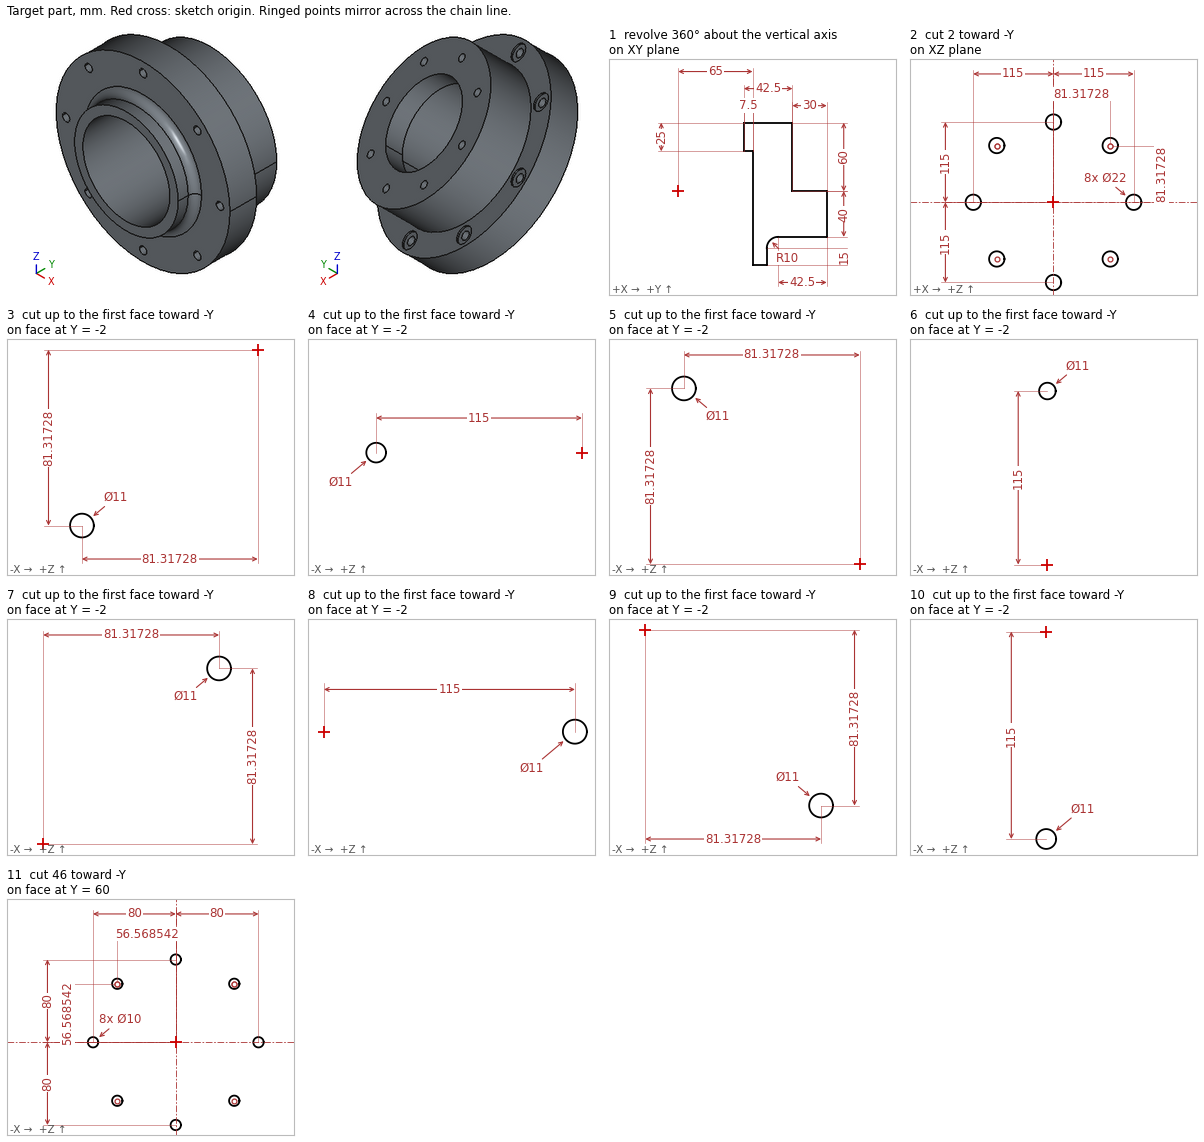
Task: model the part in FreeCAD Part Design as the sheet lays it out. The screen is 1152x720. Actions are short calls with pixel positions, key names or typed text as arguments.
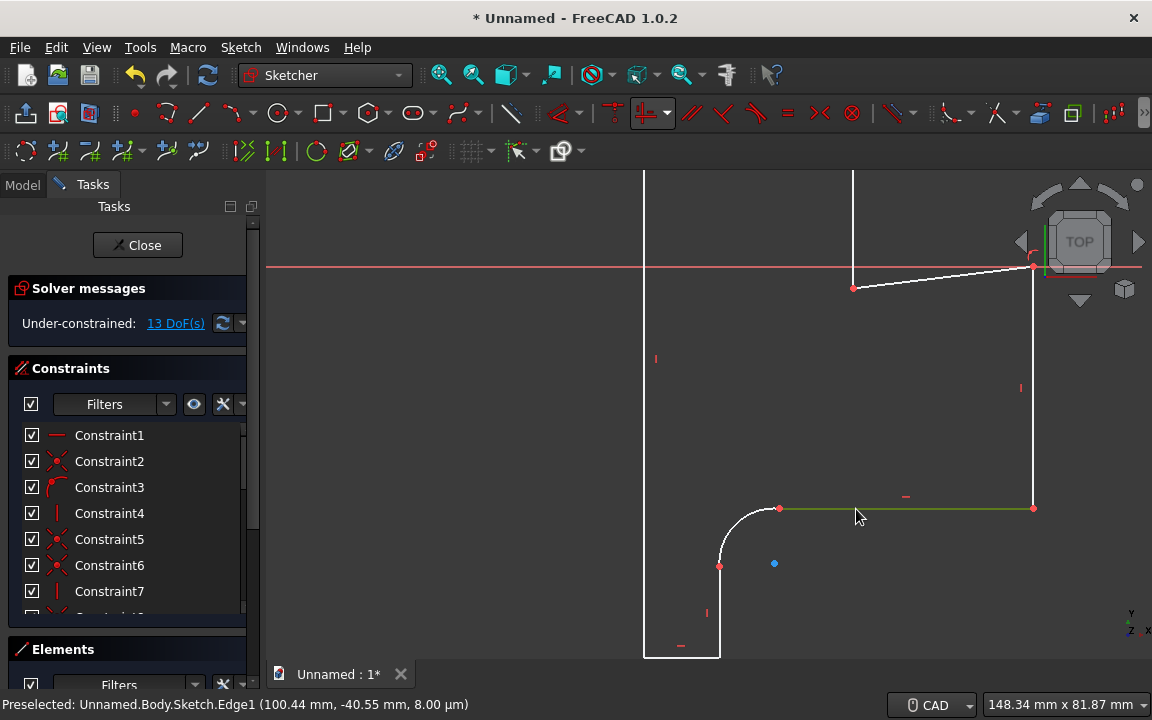
click(752, 513)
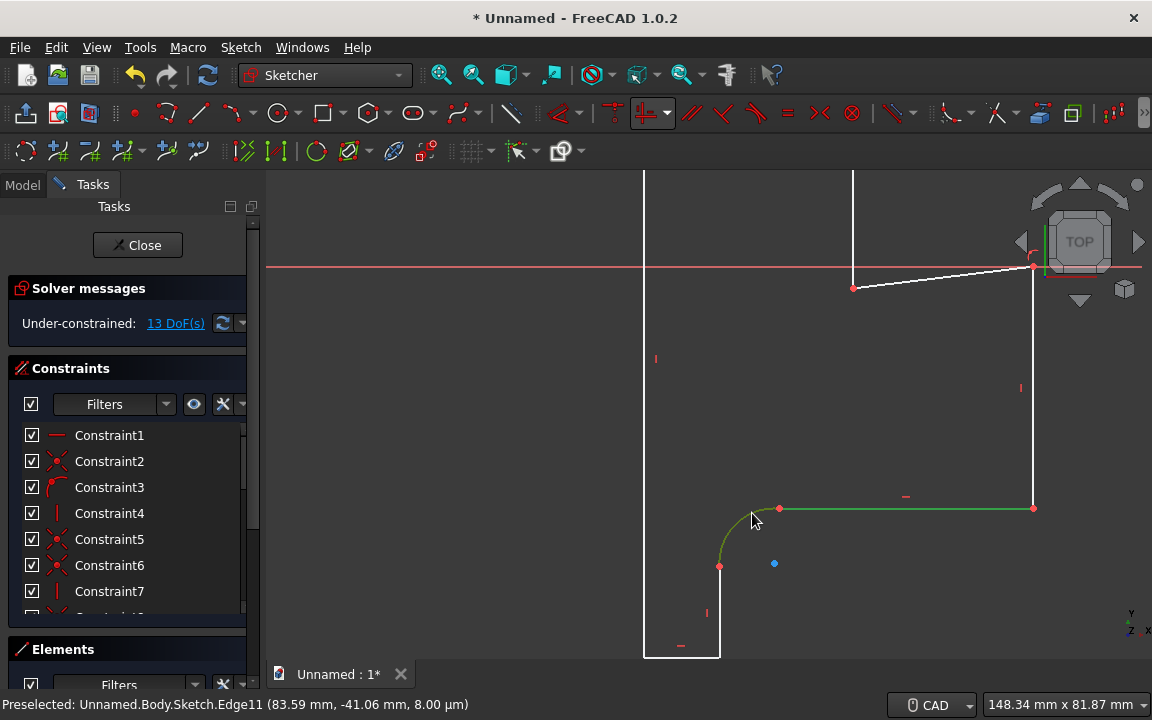
key(t)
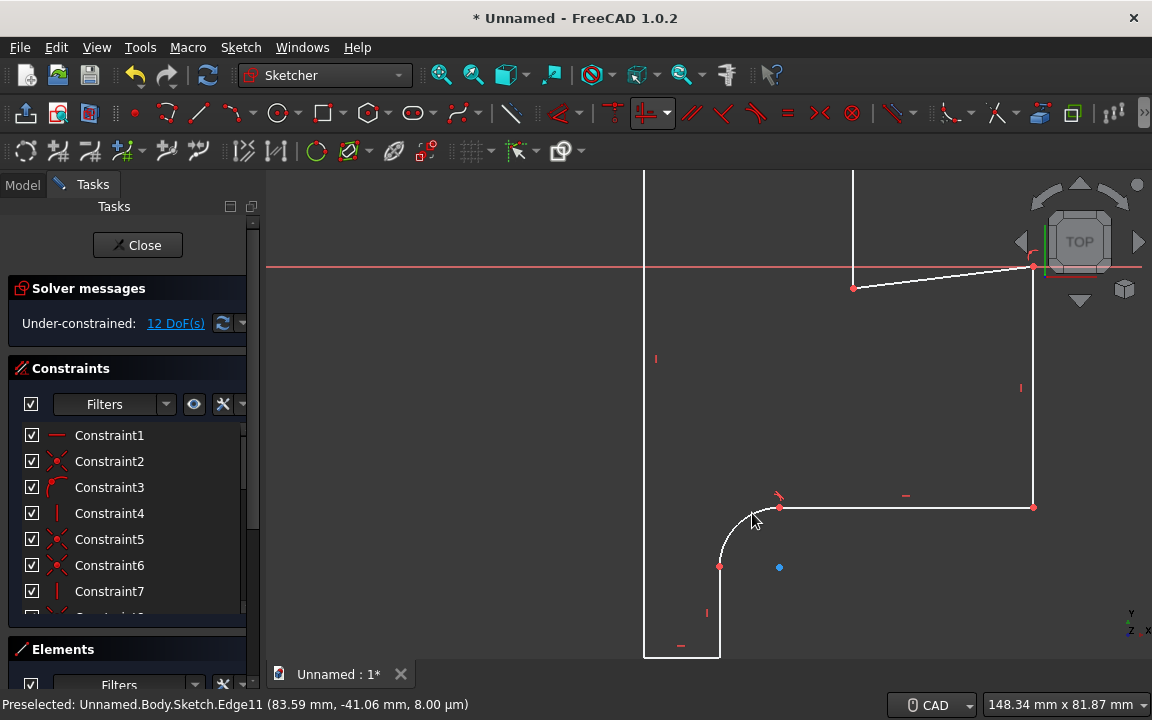
click(720, 630)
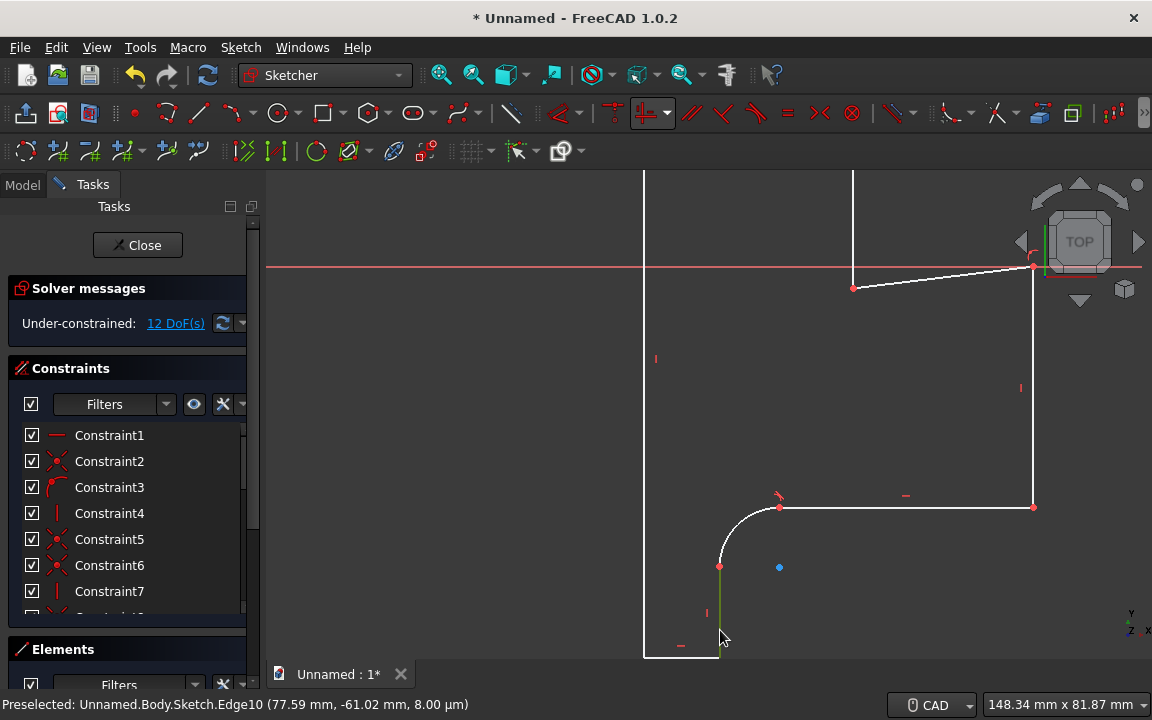
click(753, 514)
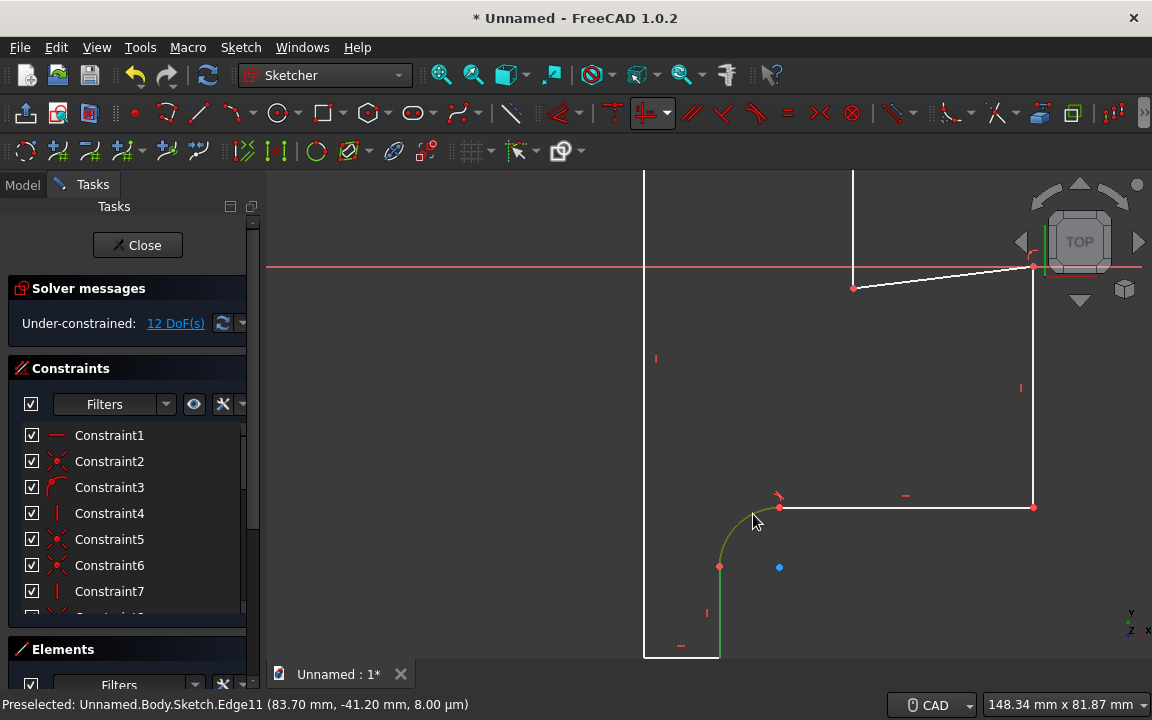
click(756, 114)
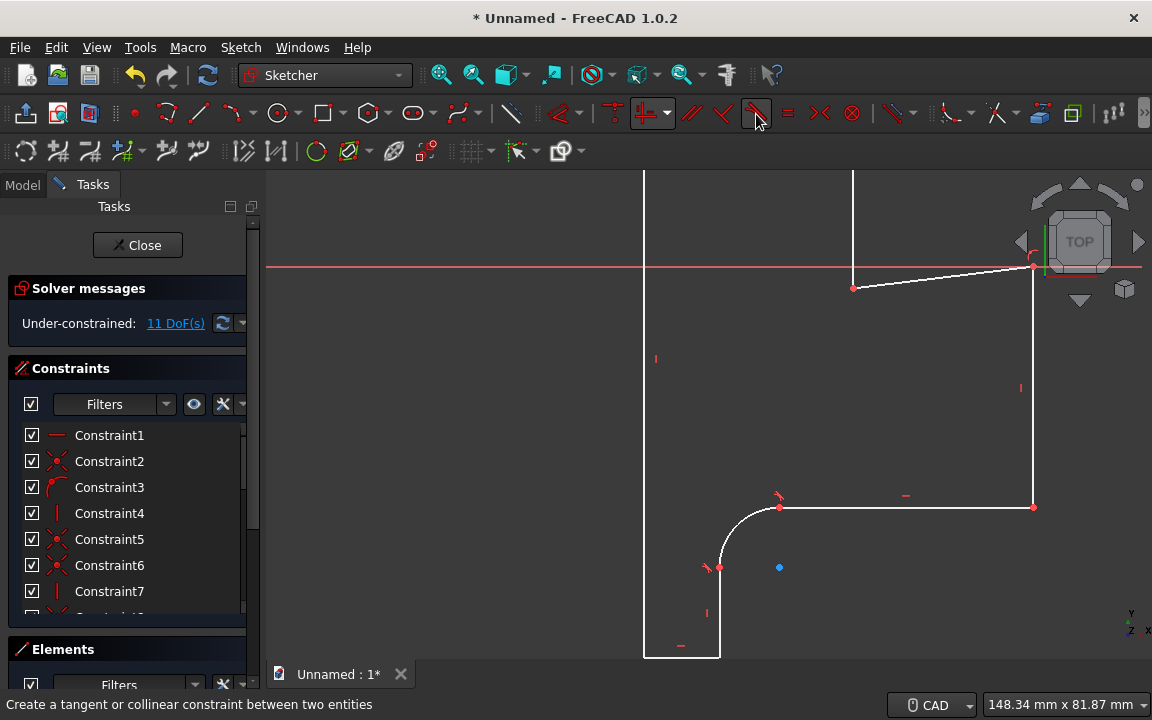
click(907, 282)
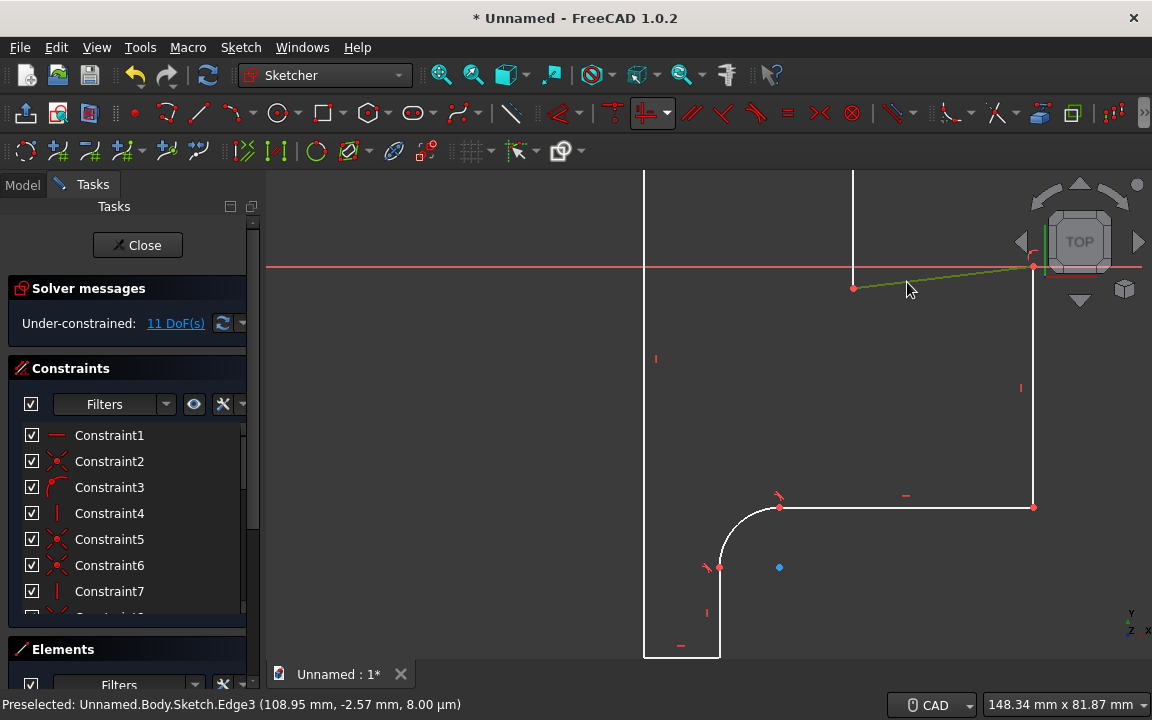
key(h)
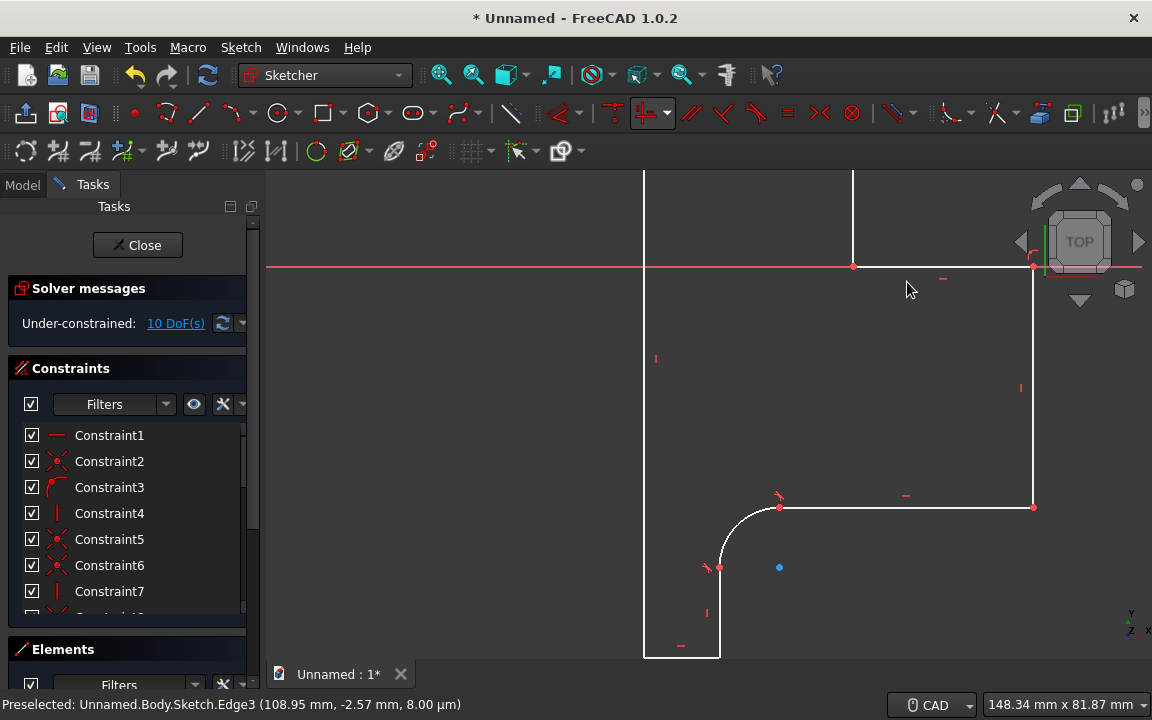
click(558, 114)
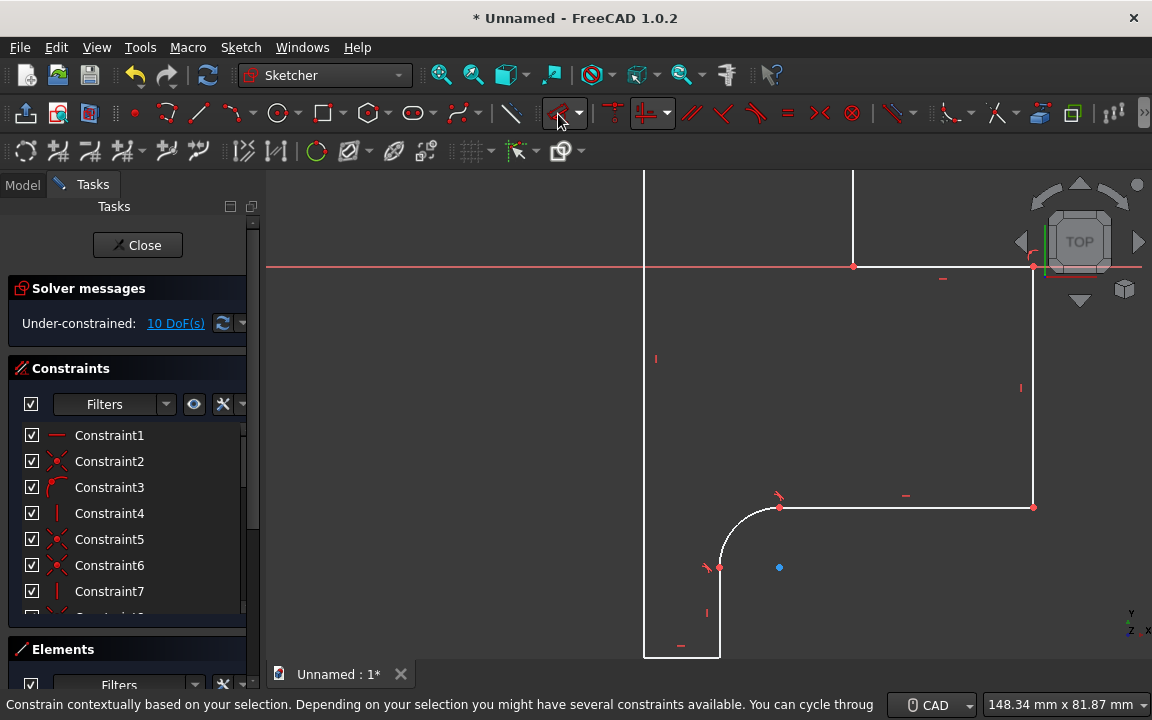
click(752, 514)
click(737, 486)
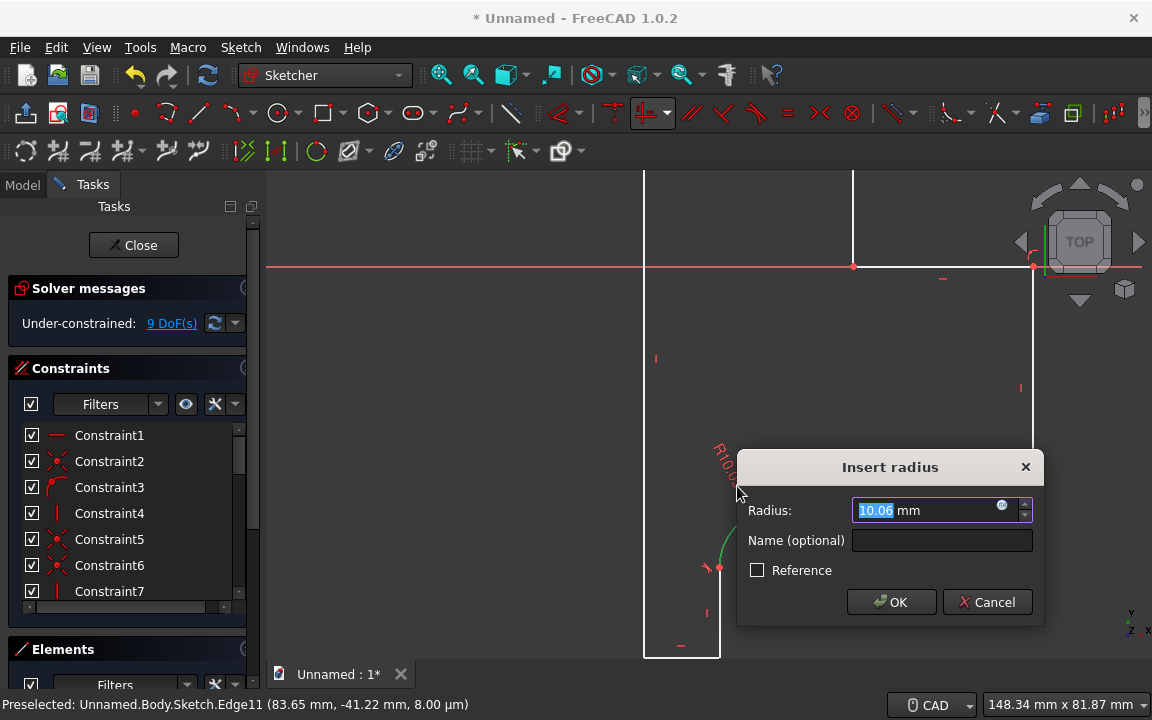
text(10)
key(Return)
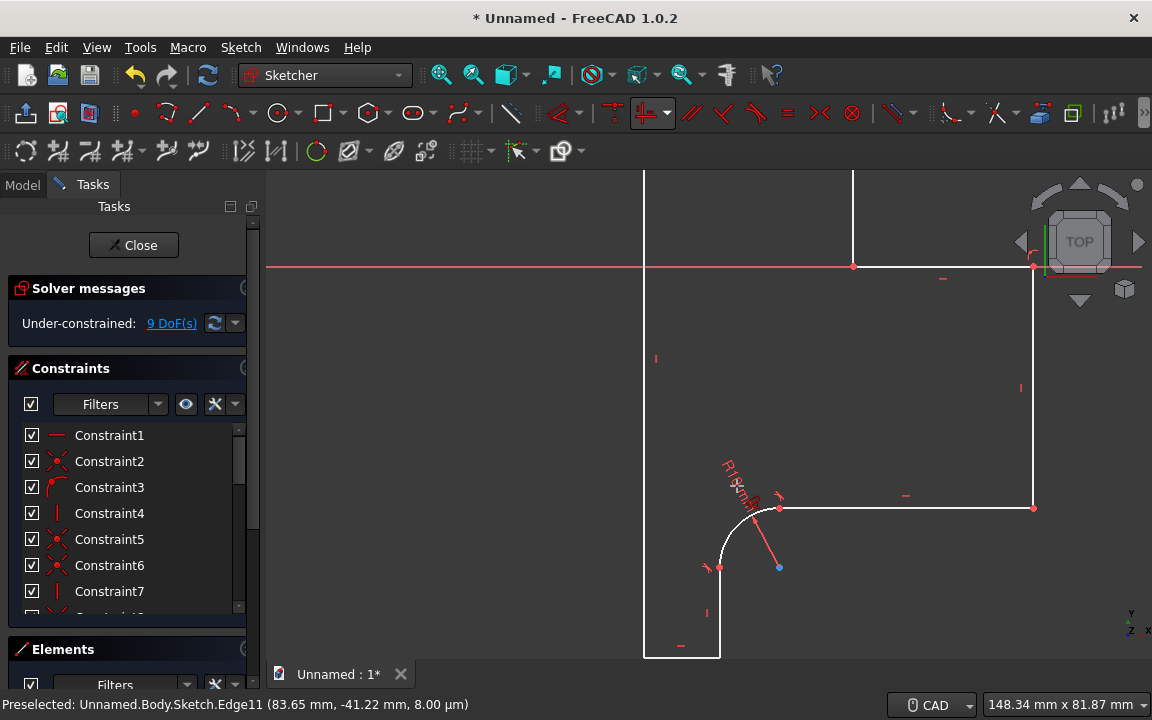
scroll(637, 523, down, 4)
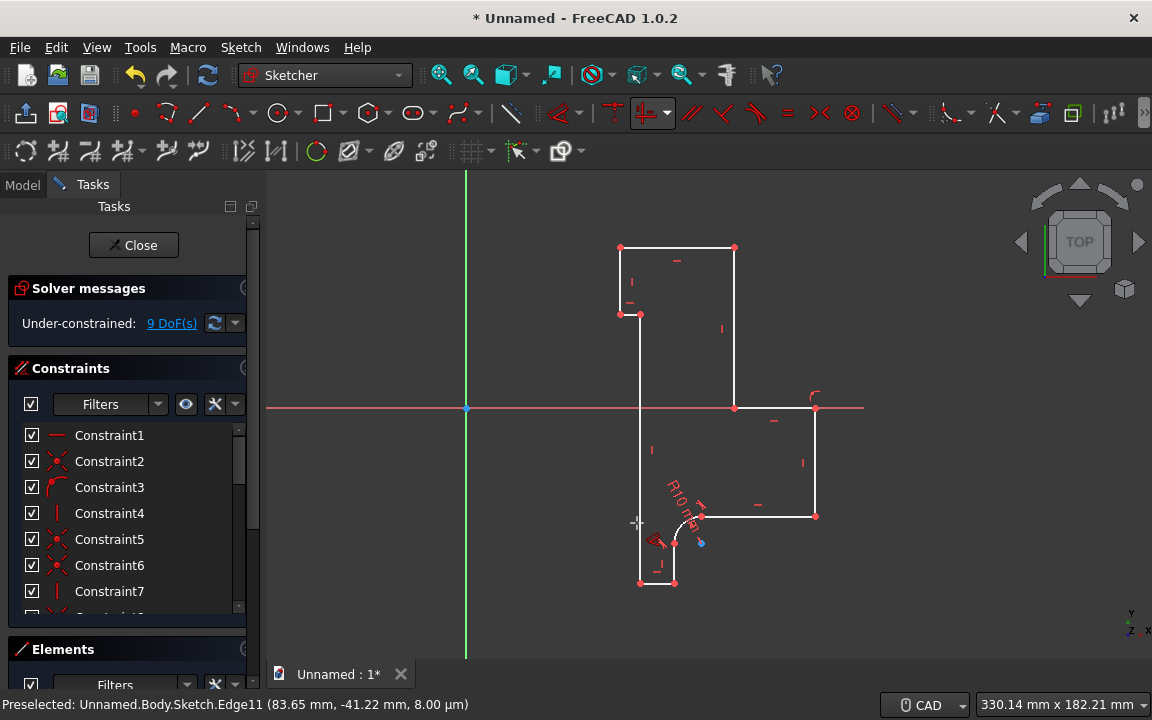
click(815, 484)
click(849, 462)